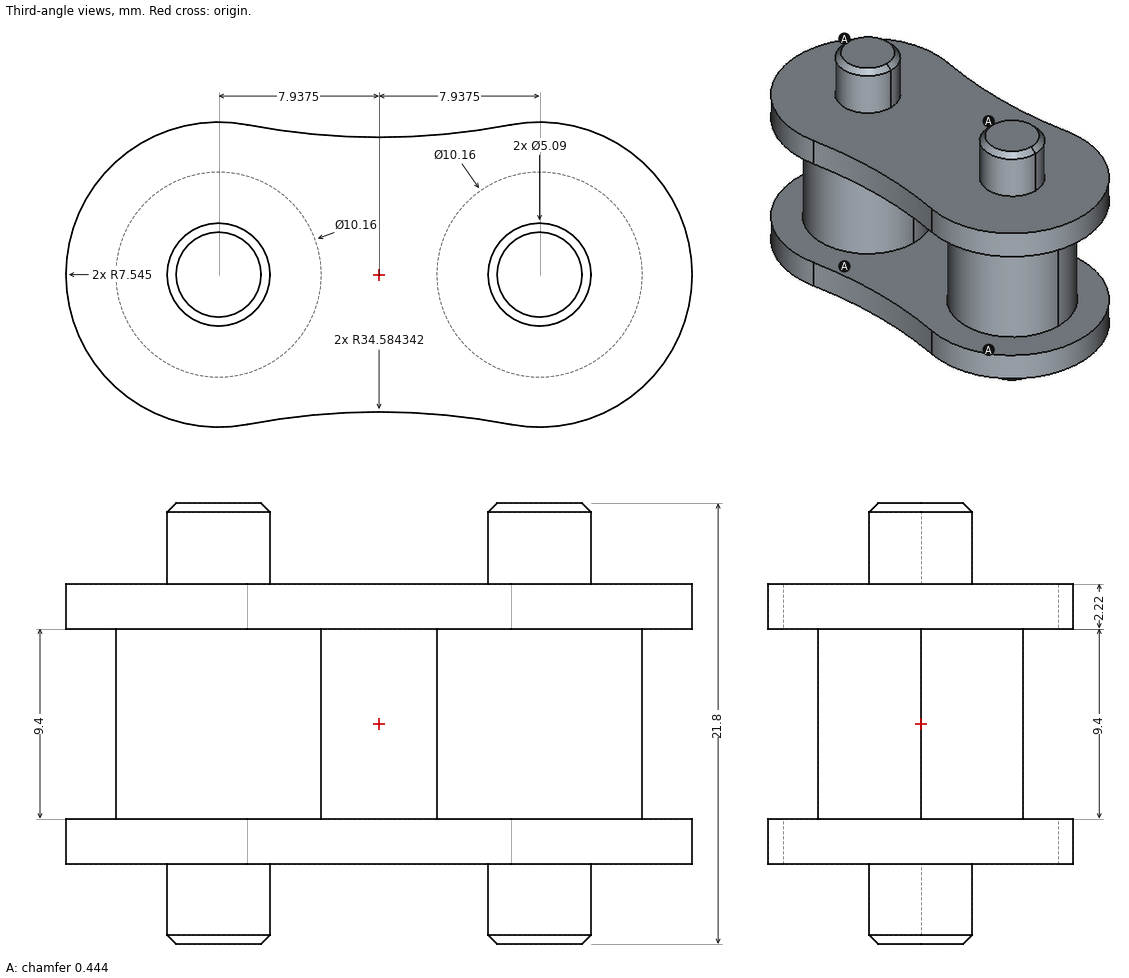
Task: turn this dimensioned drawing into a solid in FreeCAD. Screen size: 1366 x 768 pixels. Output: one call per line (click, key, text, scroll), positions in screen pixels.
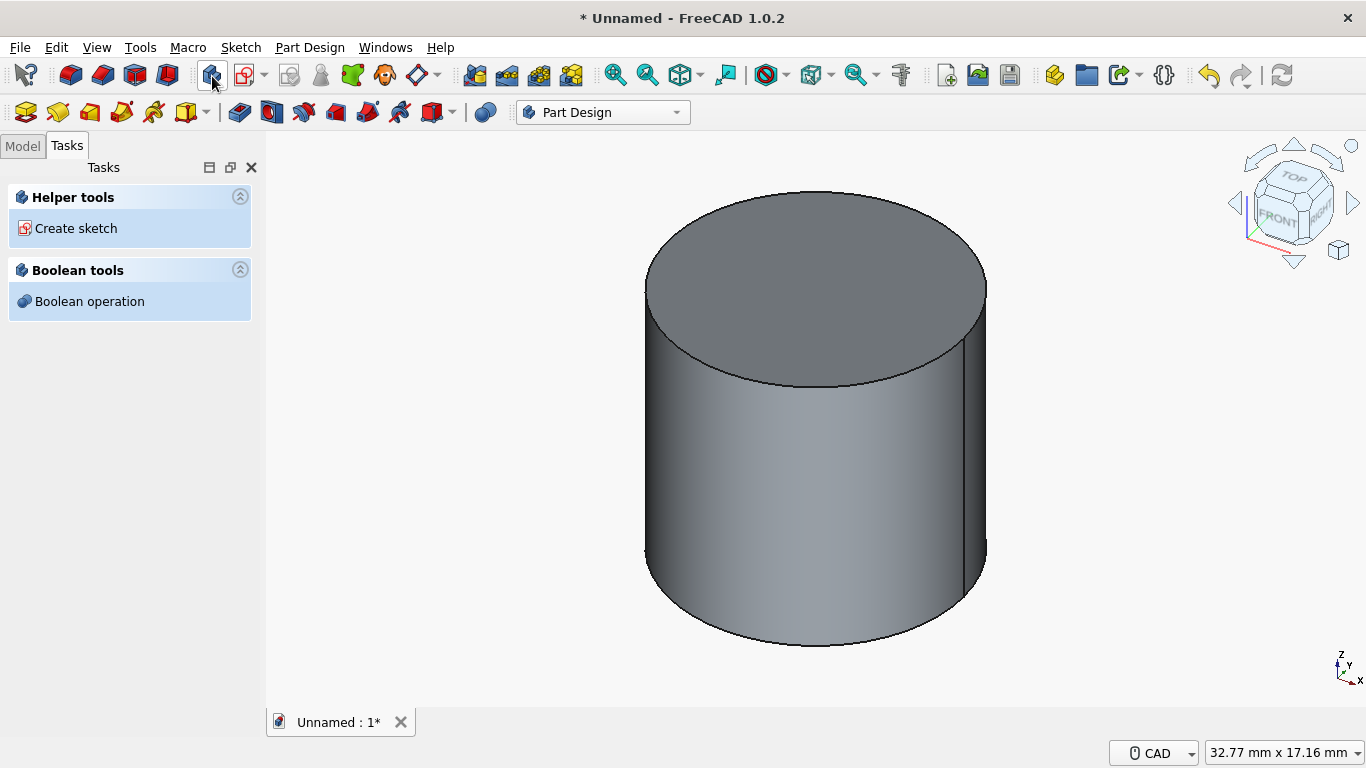
click(306, 667)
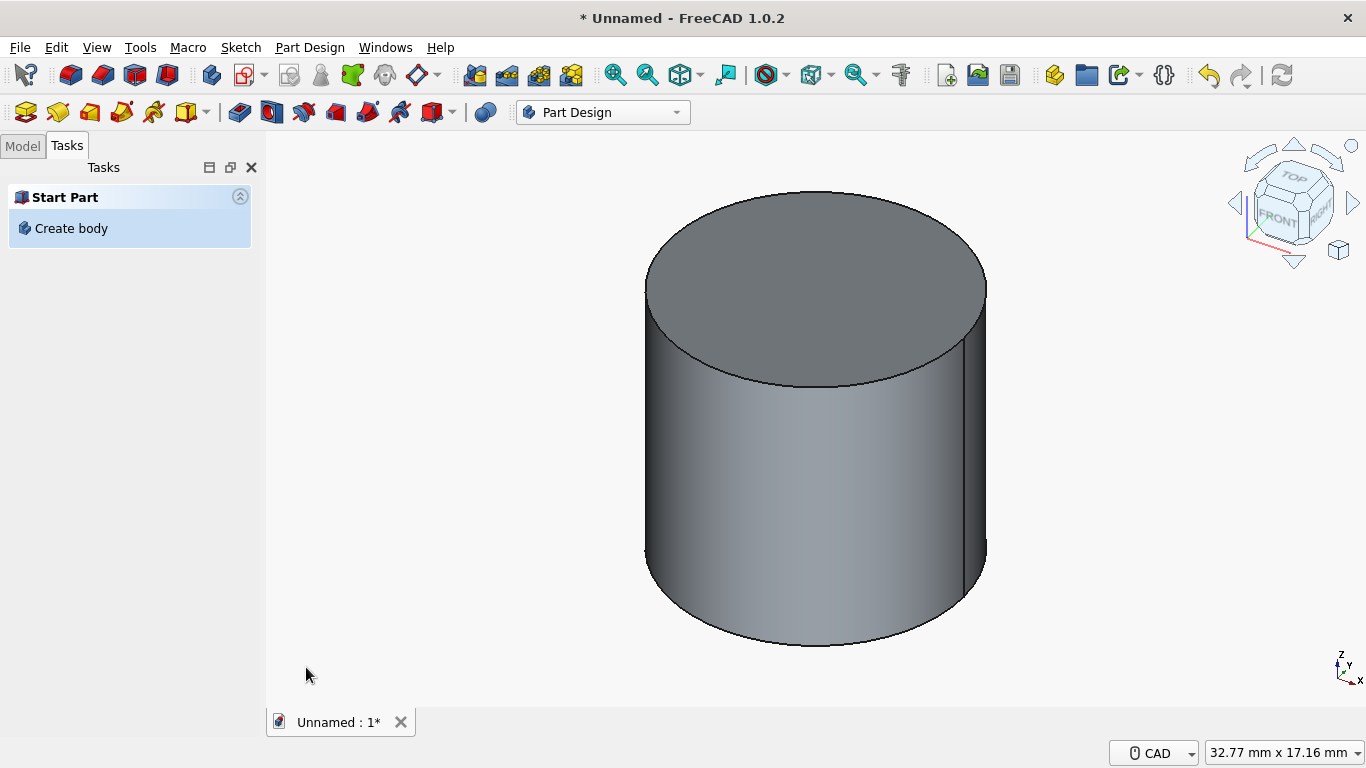
click(244, 76)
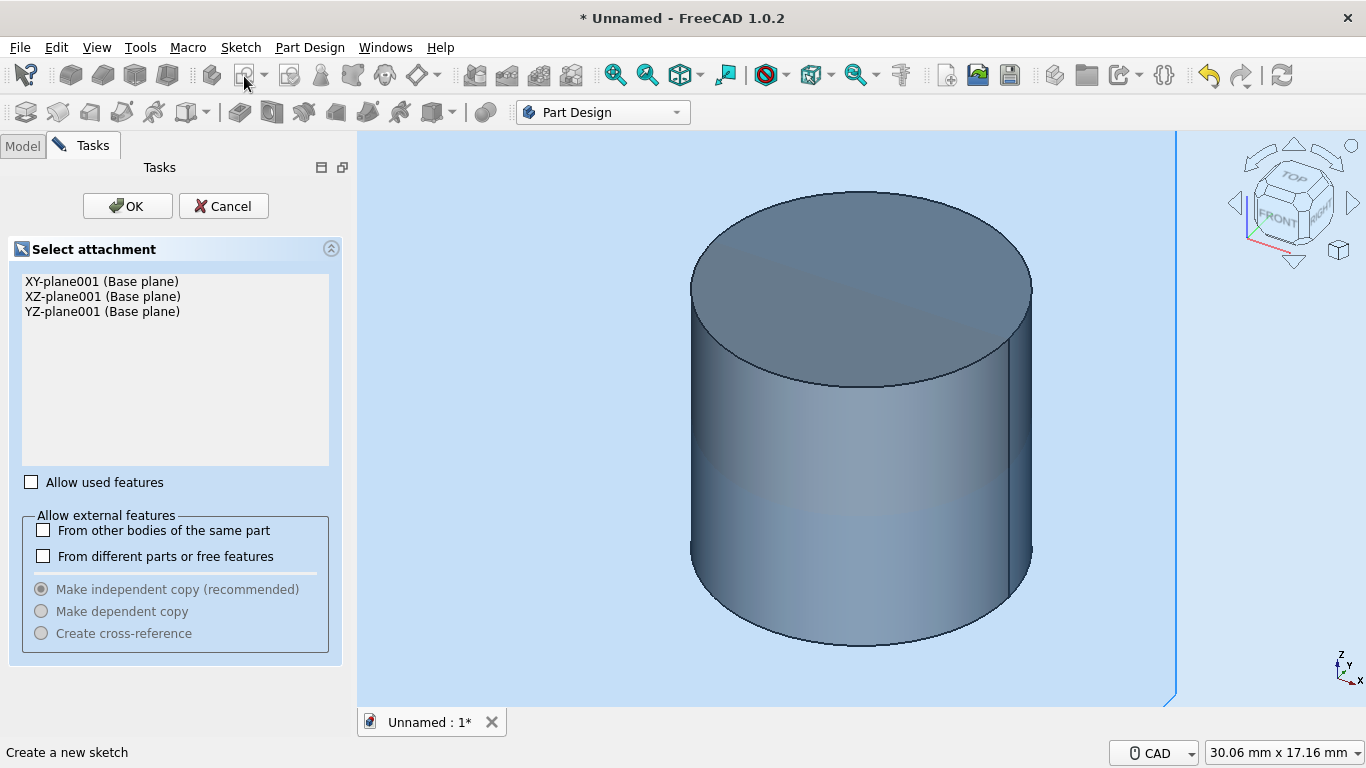
click(82, 282)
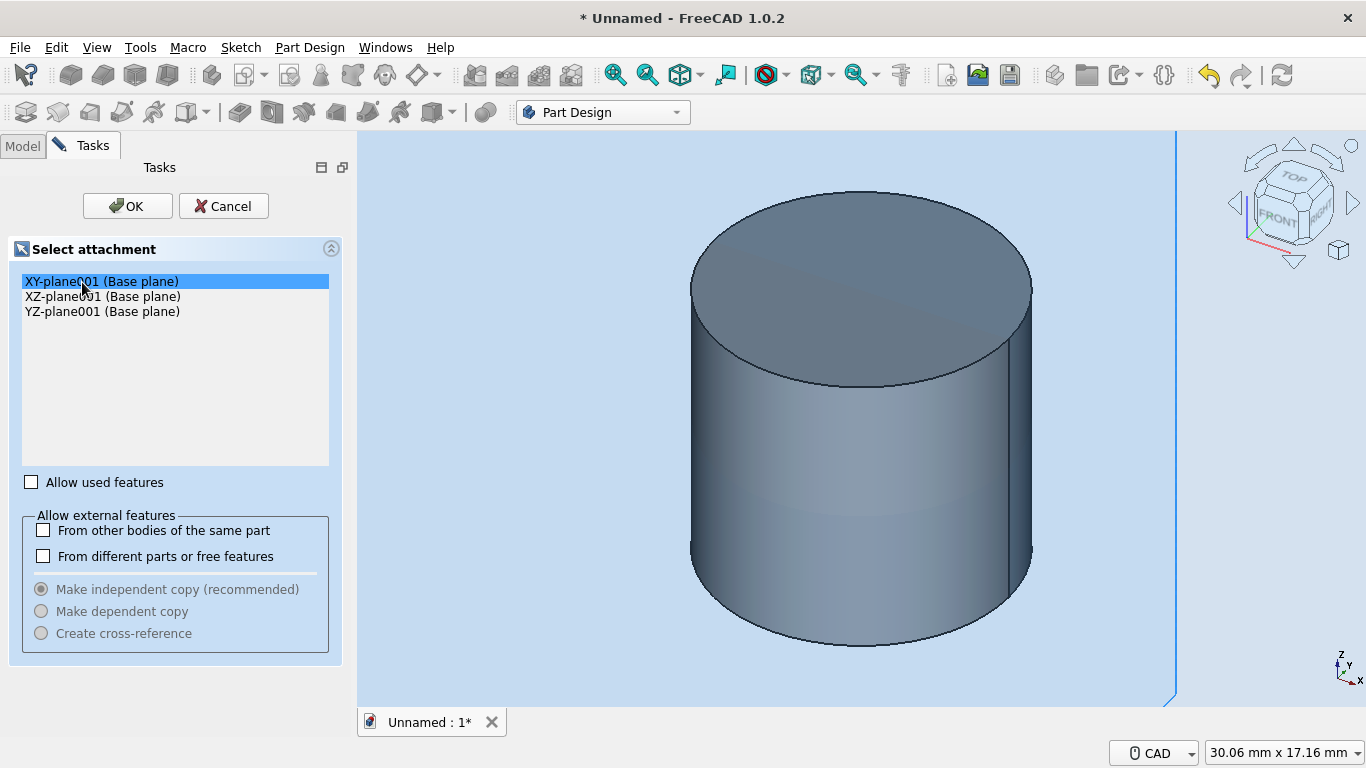
click(128, 206)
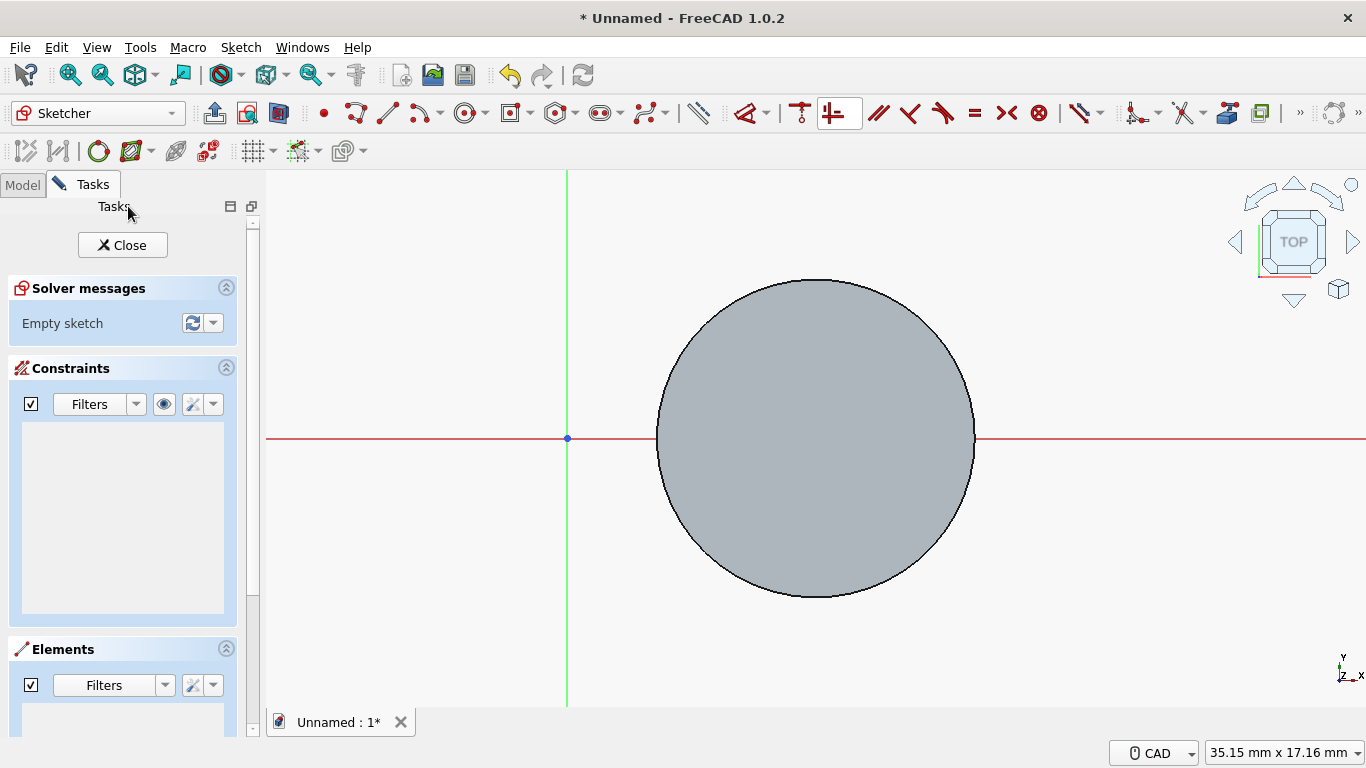
scroll(1201, 439, down, 1)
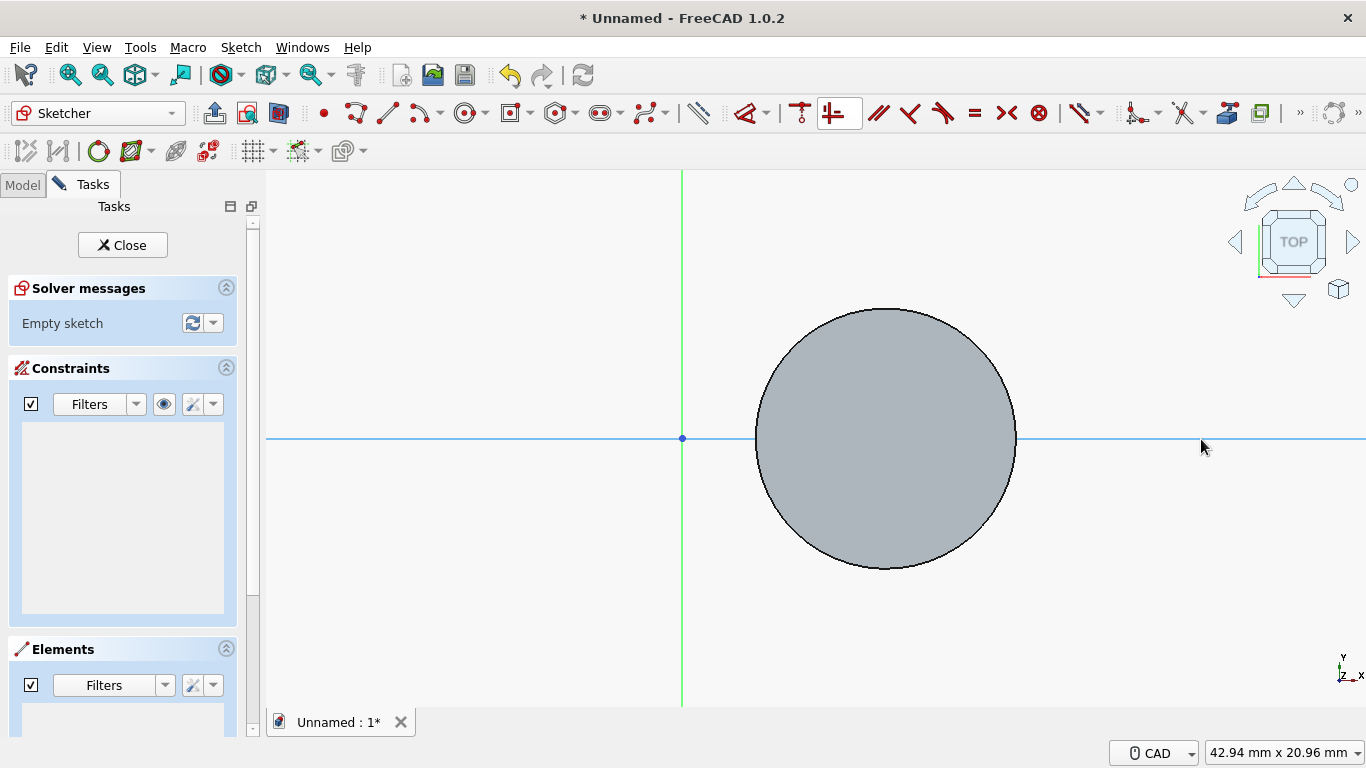
click(466, 114)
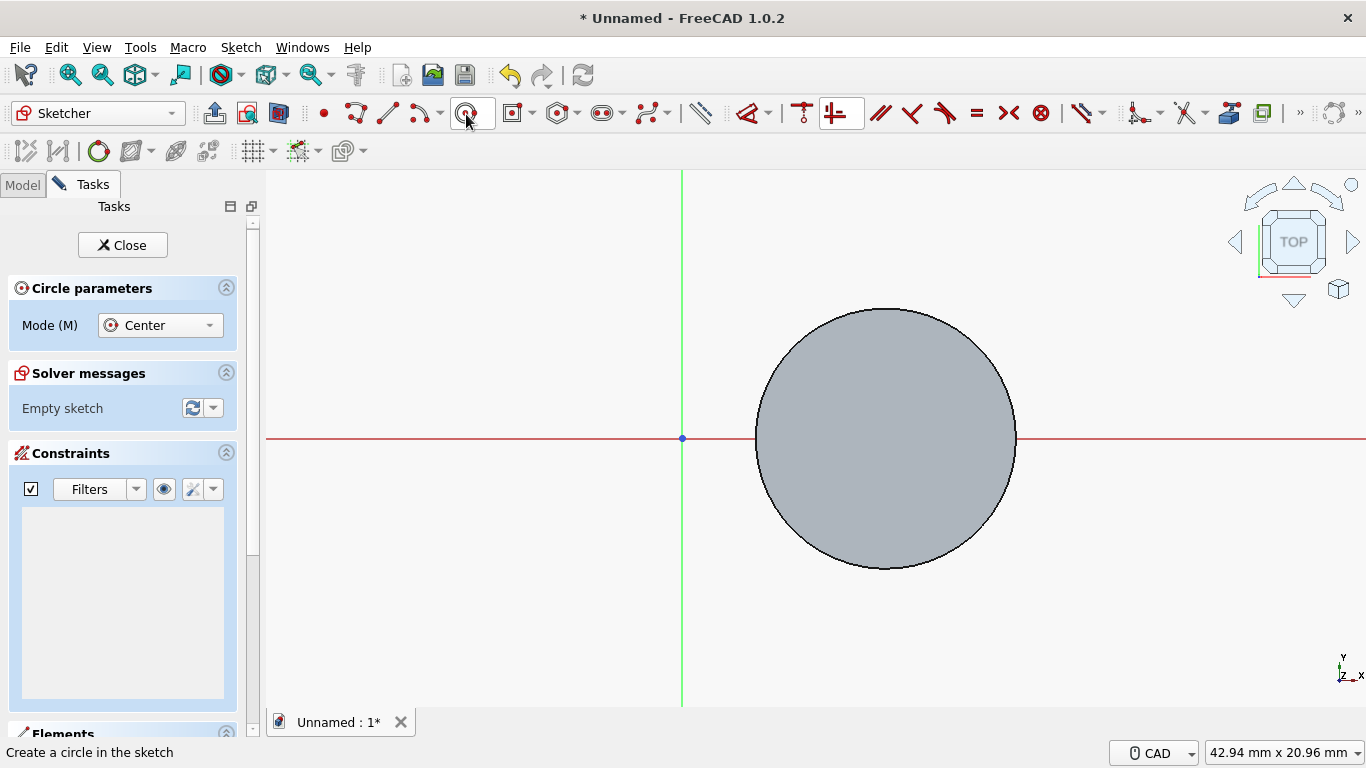
click(479, 439)
move(571, 347)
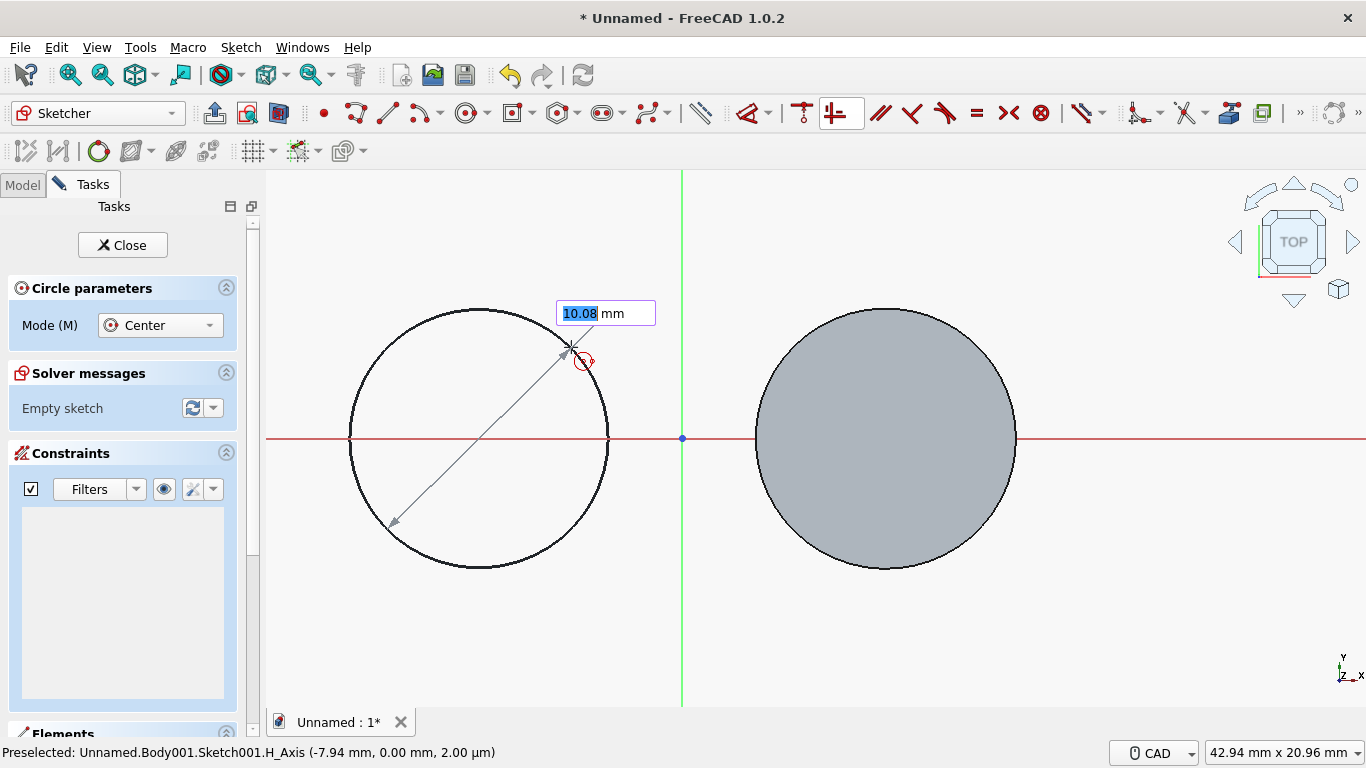
text(10.16)
key(Return)
key(Escape)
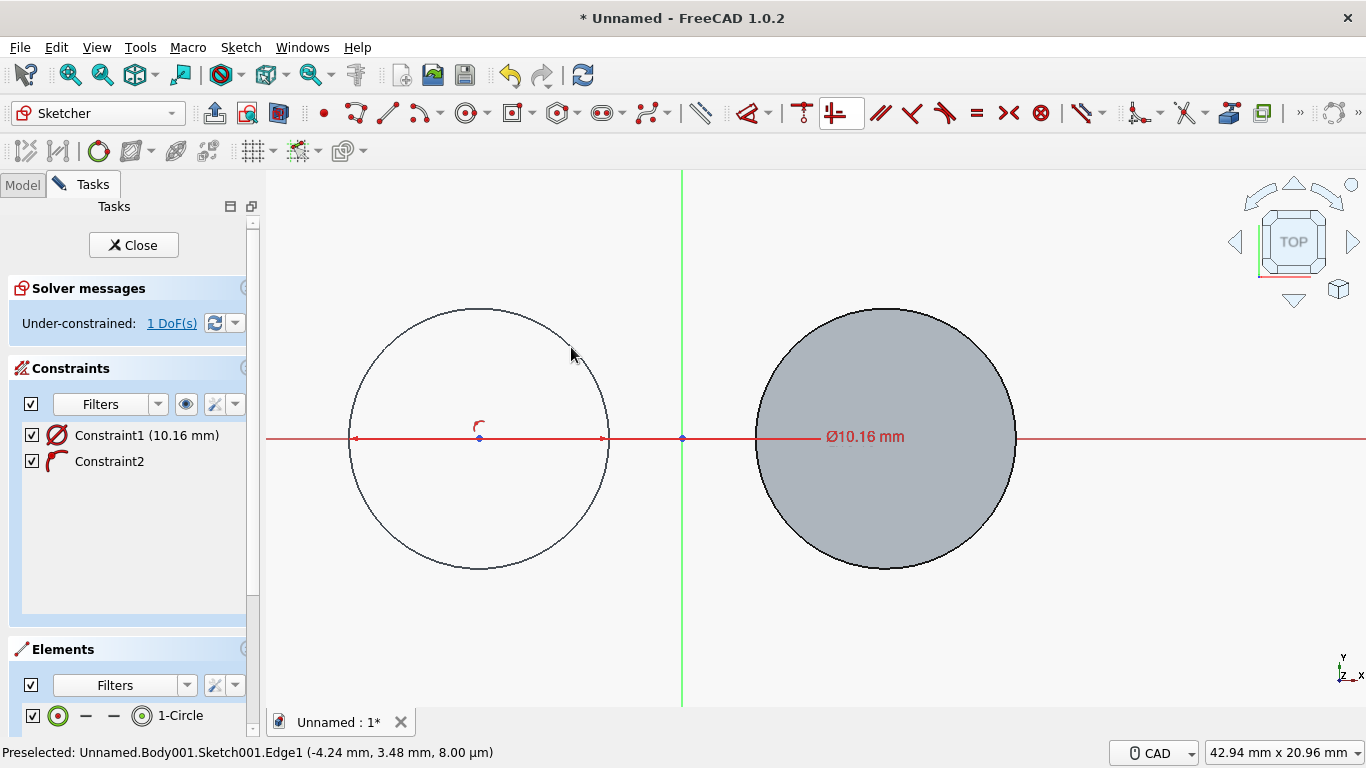
click(748, 114)